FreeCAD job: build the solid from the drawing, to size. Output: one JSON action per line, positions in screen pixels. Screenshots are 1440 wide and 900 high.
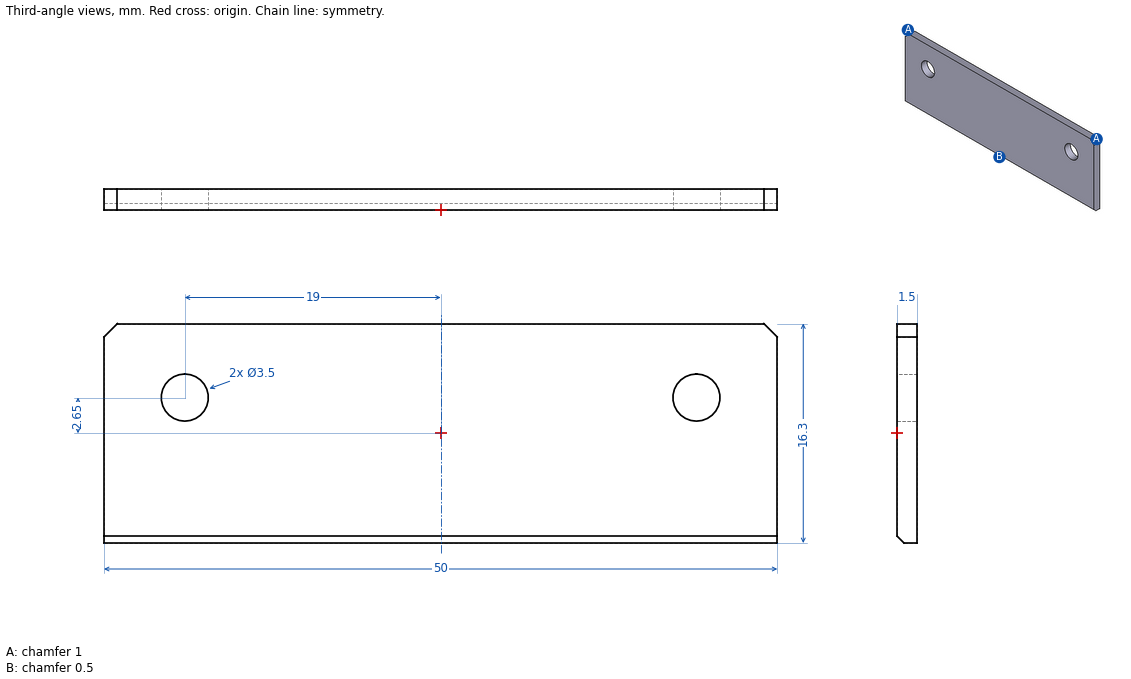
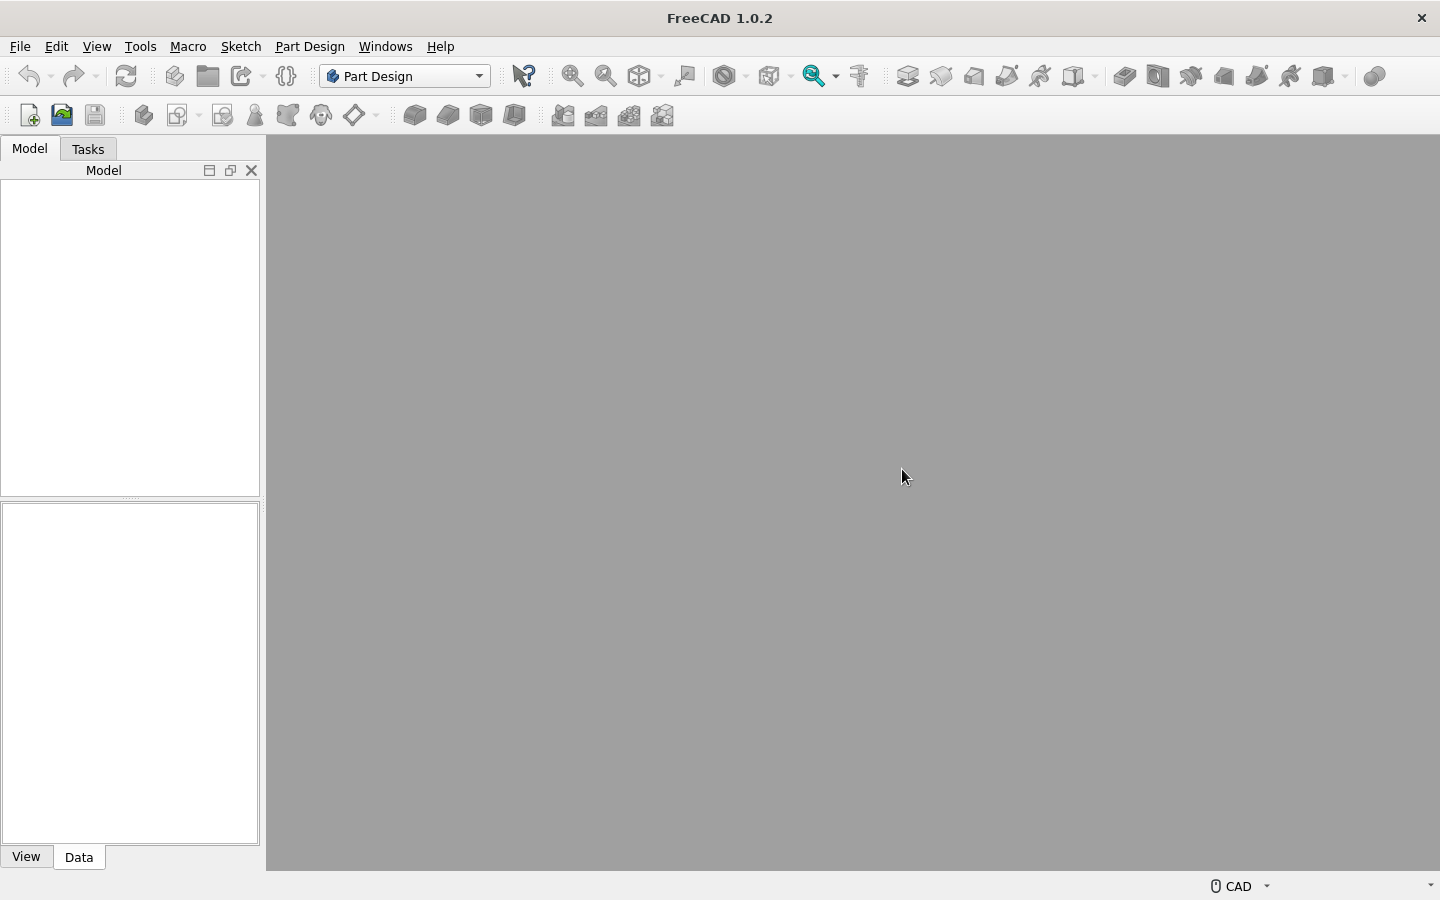
{"action": "left_click", "coordinate": [29, 116]}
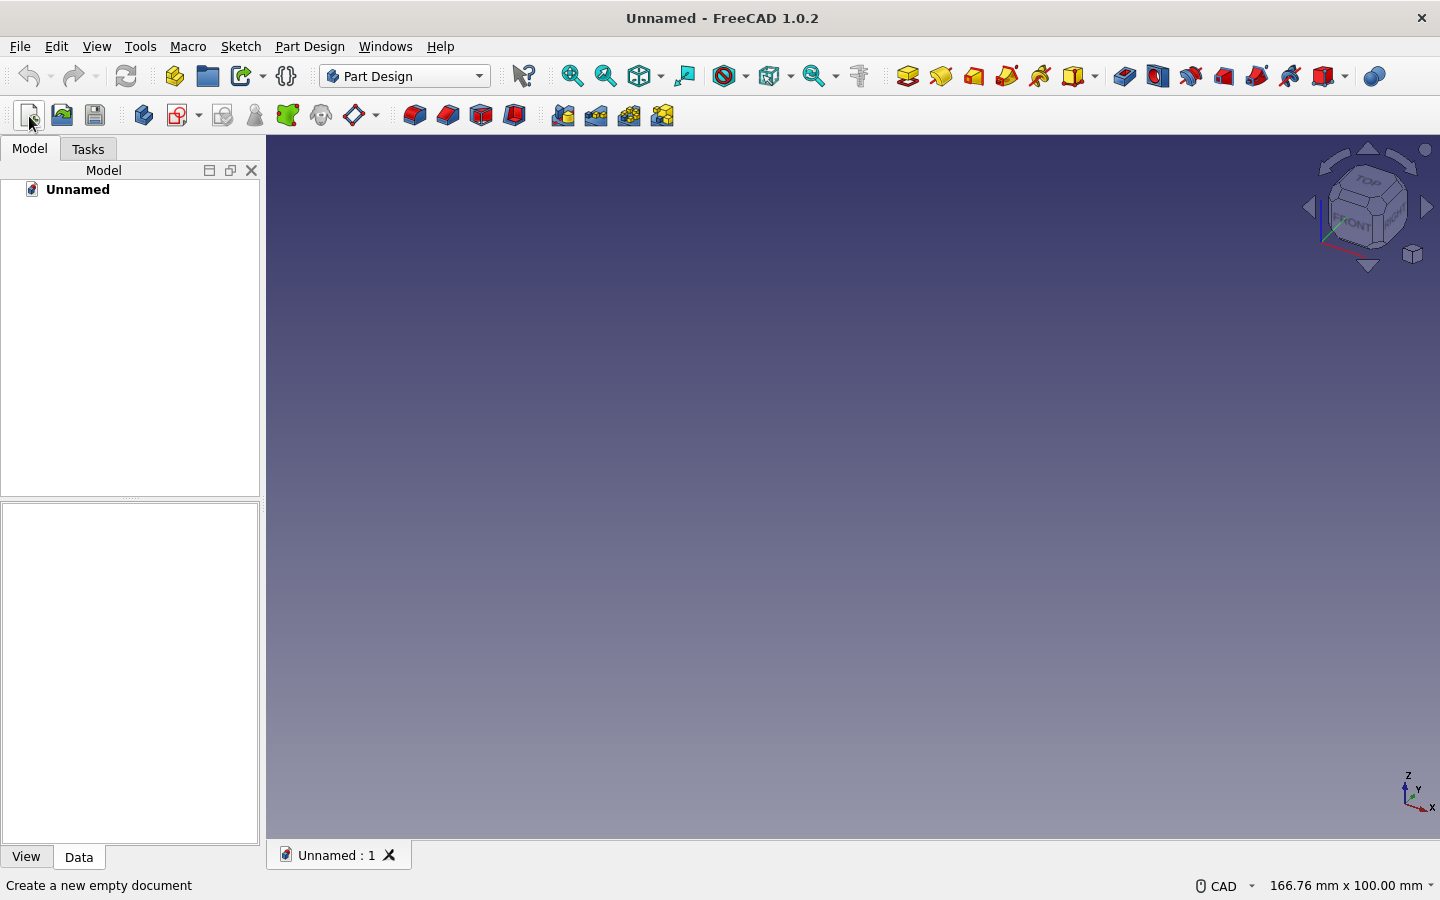
{"action": "left_click", "coordinate": [176, 116]}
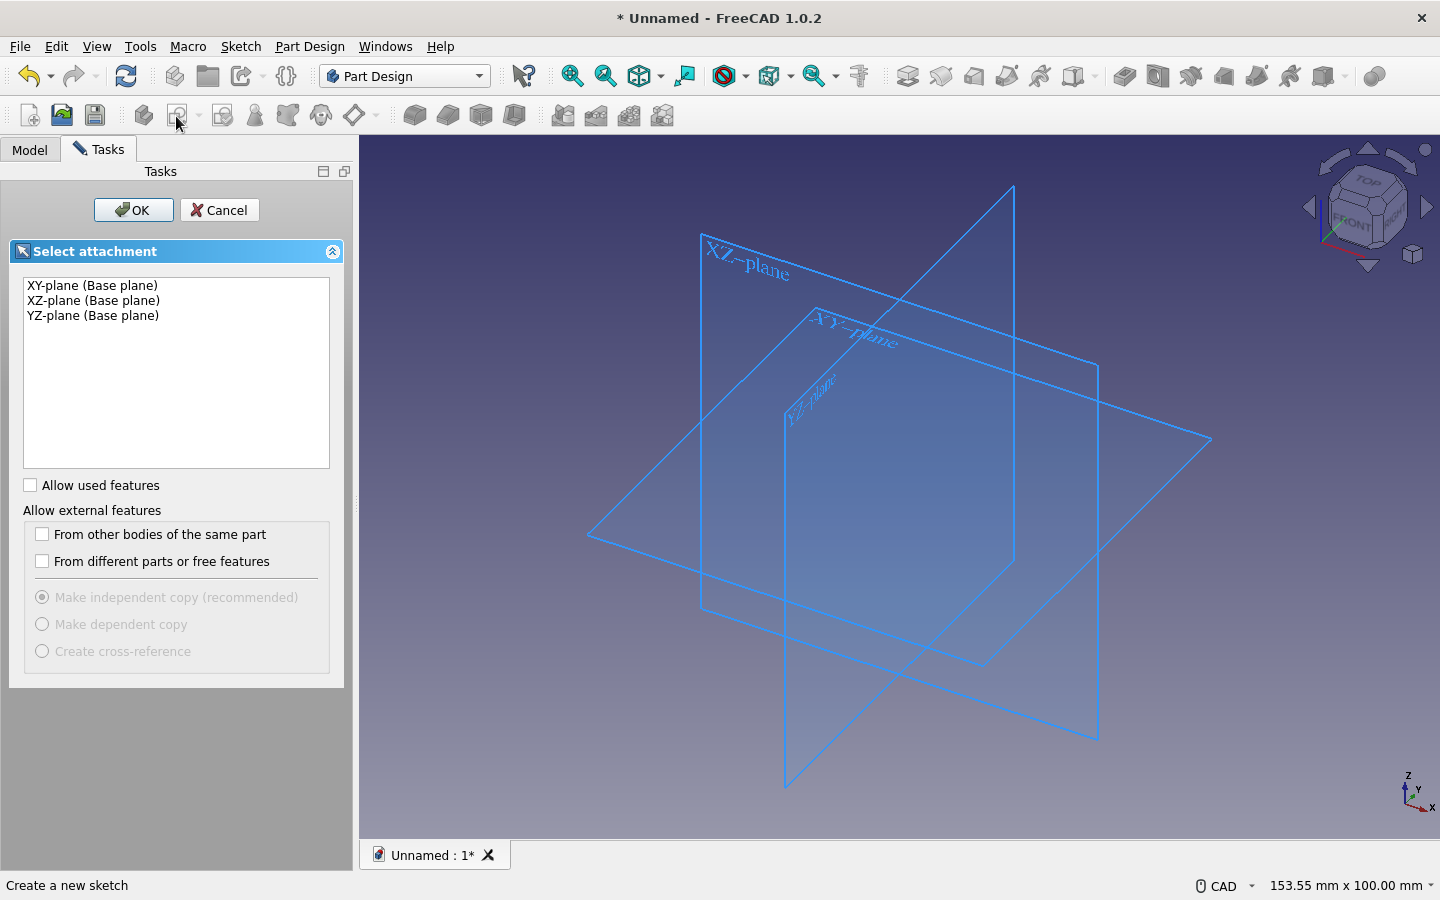
{"action": "left_click", "coordinate": [84, 300]}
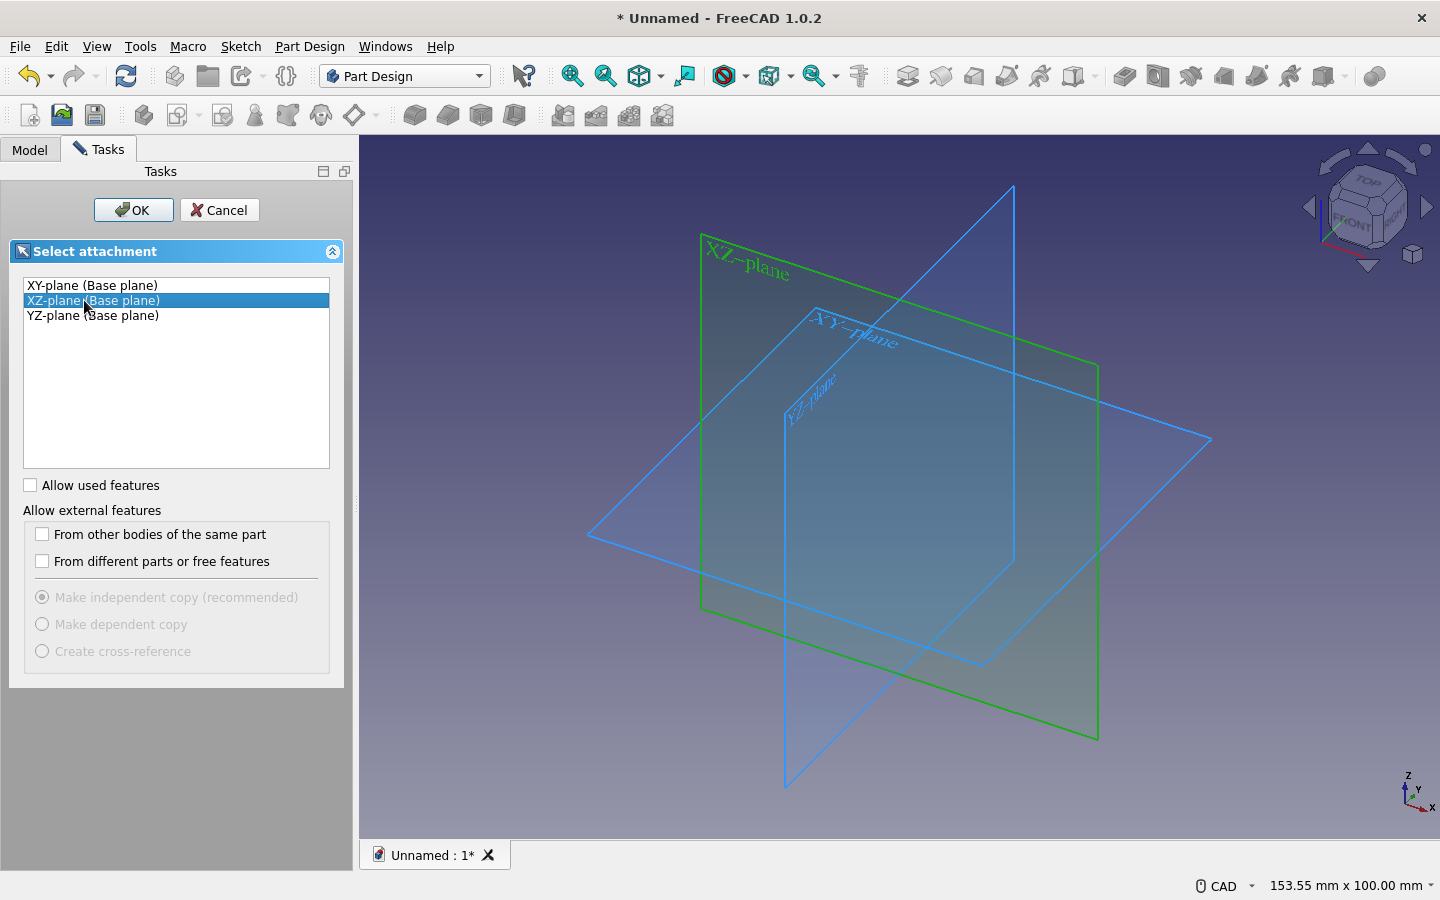
{"action": "left_click", "coordinate": [134, 210]}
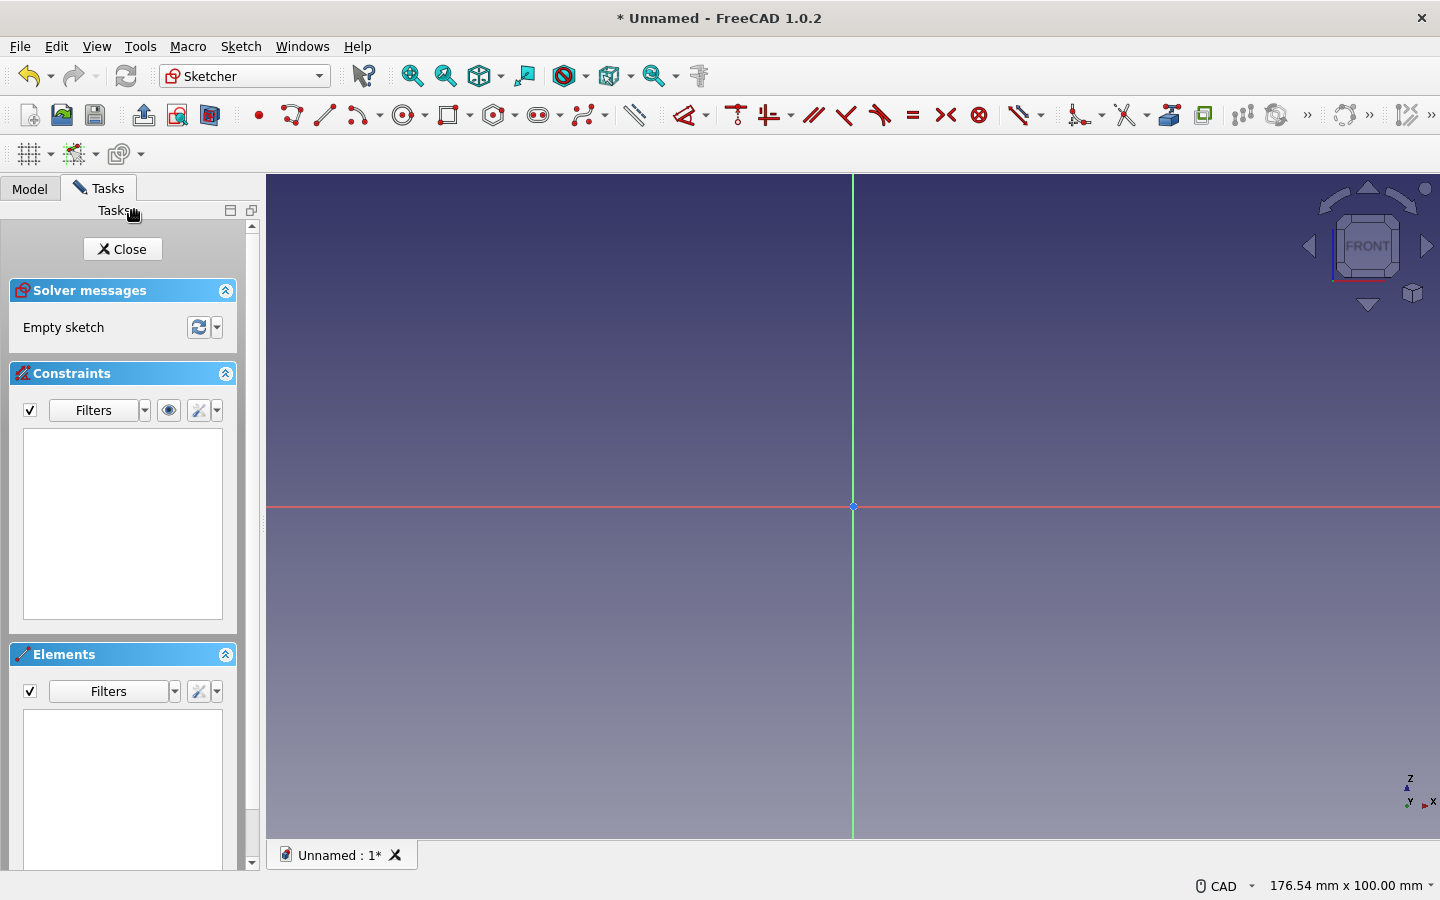
{"action": "scroll", "coordinate": [909, 506], "scroll_direction": "up", "scroll_amount": 4}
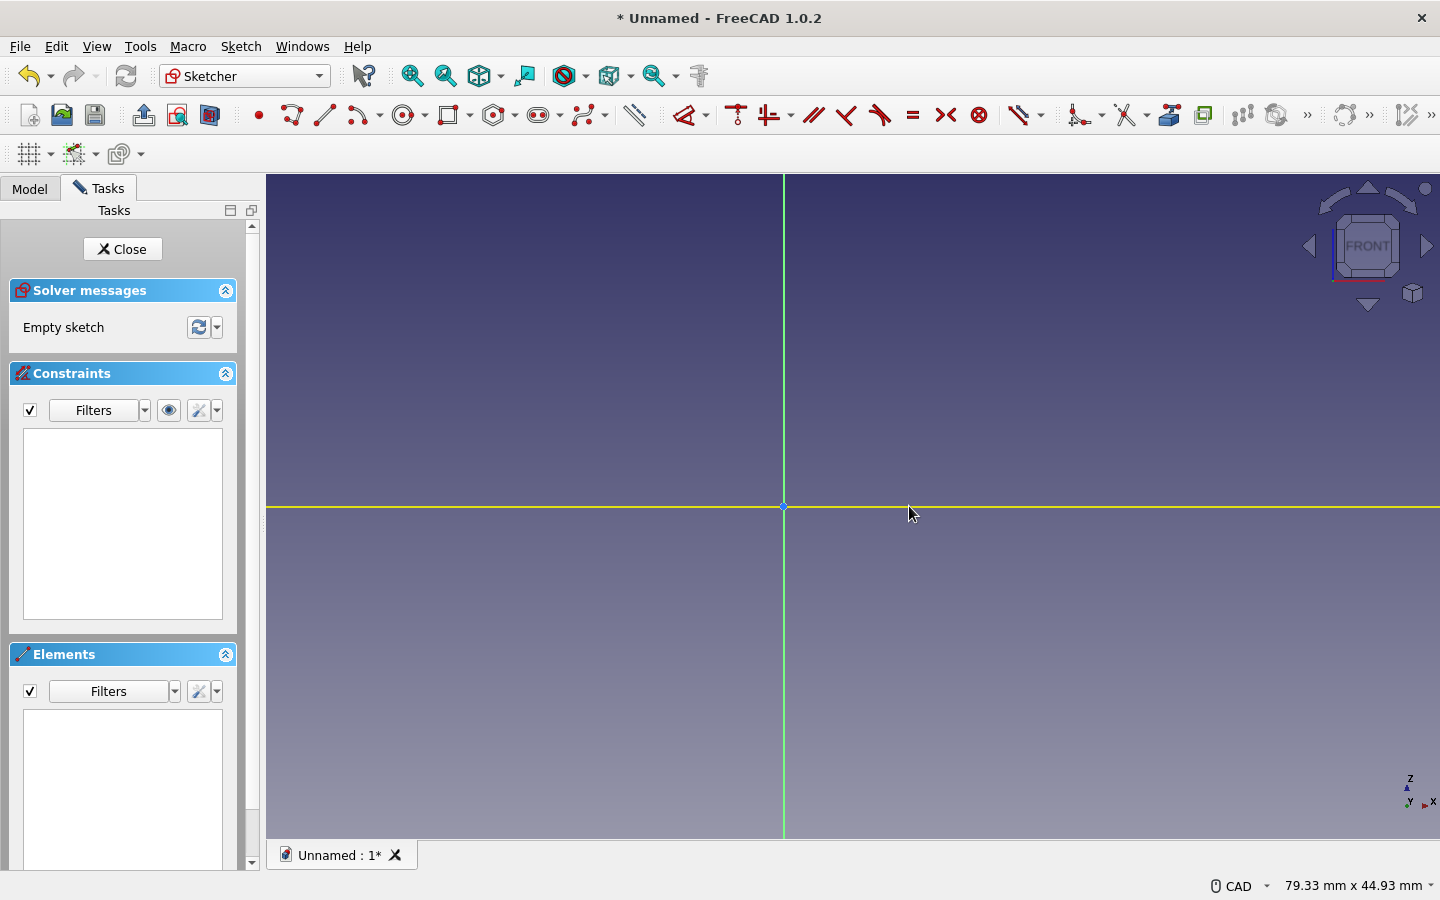
{"action": "key", "text": "g v"}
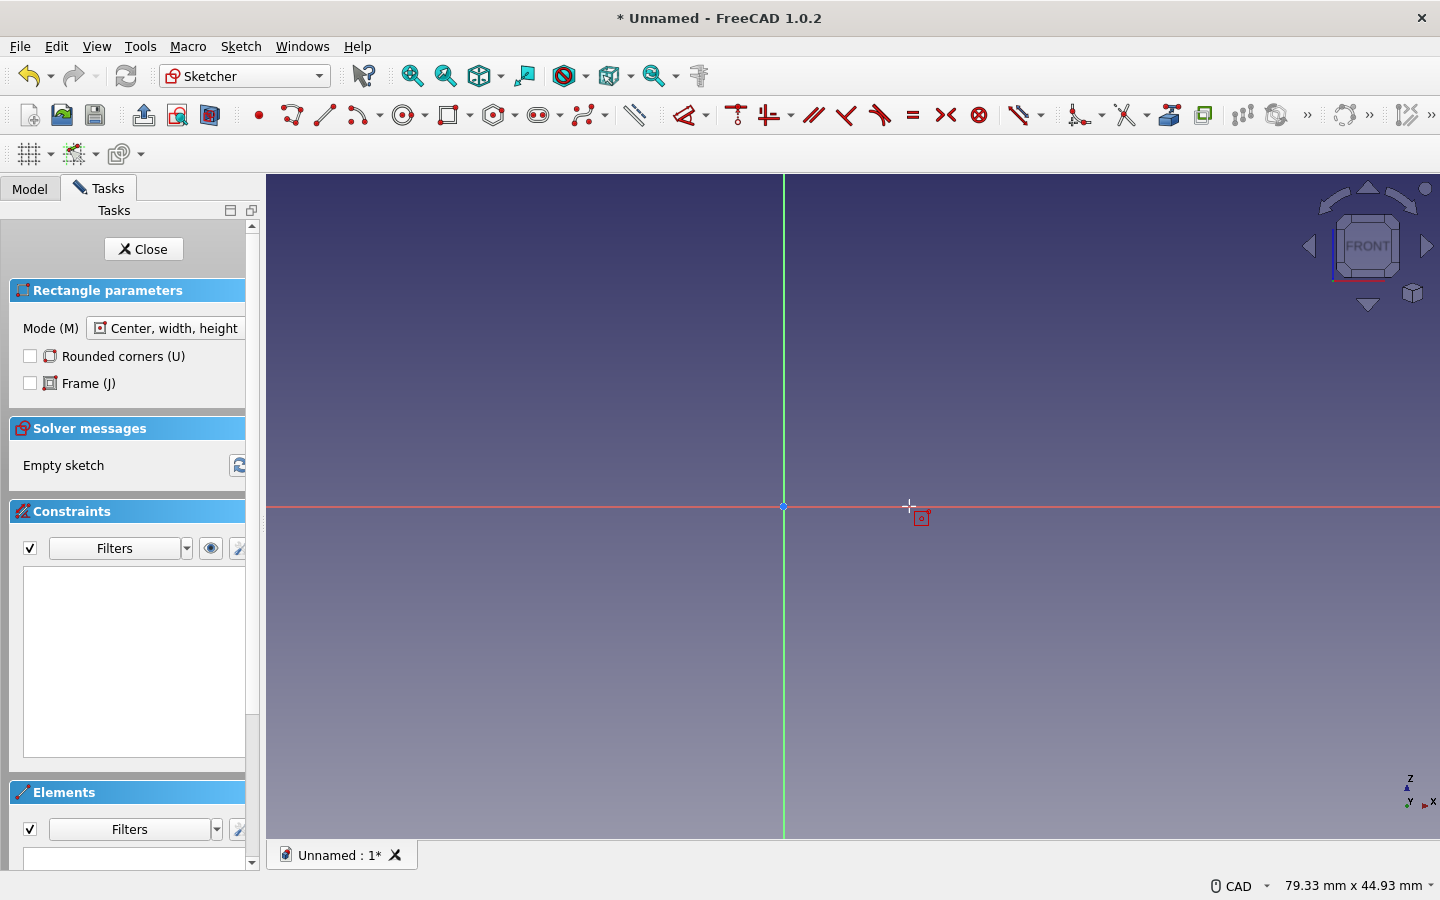
{"action": "left_click", "coordinate": [784, 506]}
{"action": "mouse_move", "coordinate": [1154, 386]}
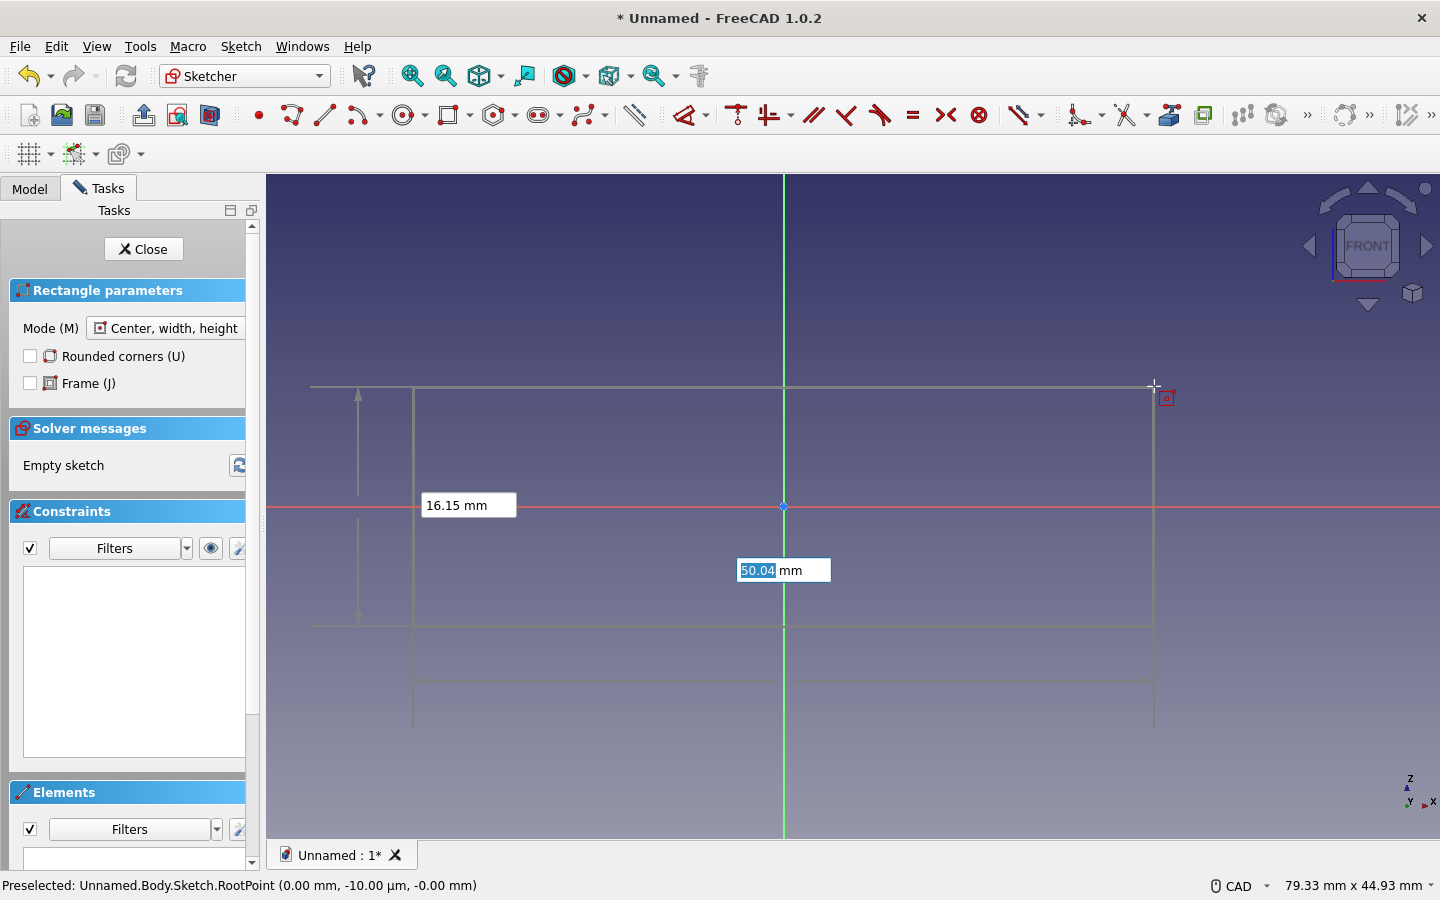
{"action": "type", "text": "50"}
{"action": "key", "text": "Tab"}
{"action": "type", "text": "16.3"}
{"action": "key", "text": "Return"}
{"action": "key", "text": "Escape"}